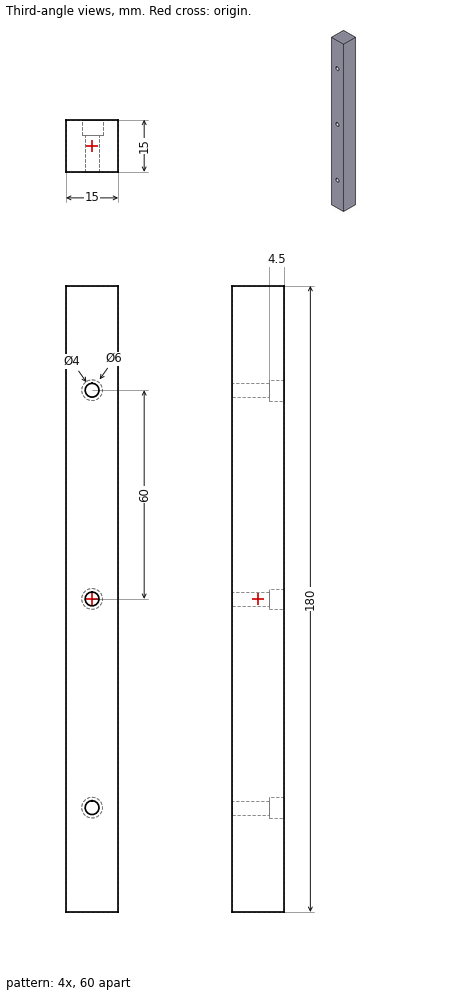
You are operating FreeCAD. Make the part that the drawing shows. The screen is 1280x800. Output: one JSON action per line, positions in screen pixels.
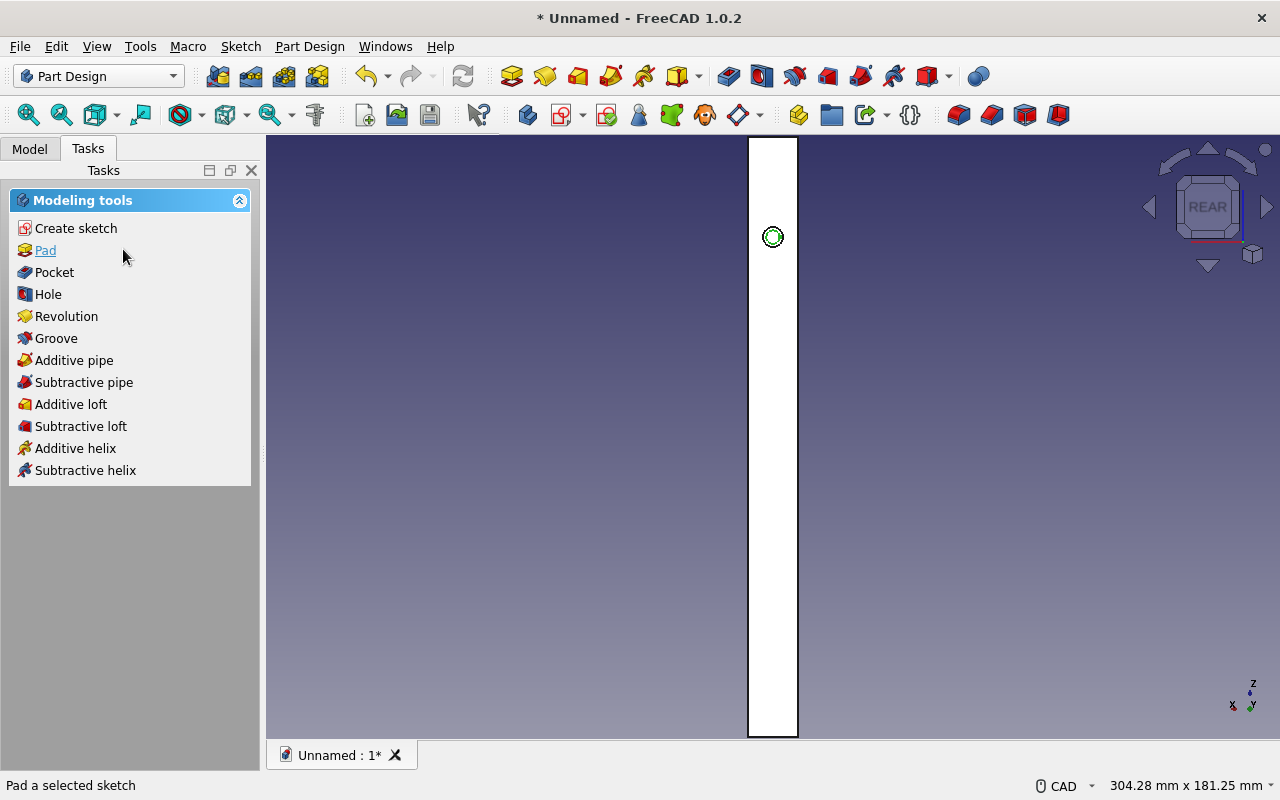
{"action": "left_click", "coordinate": [729, 76]}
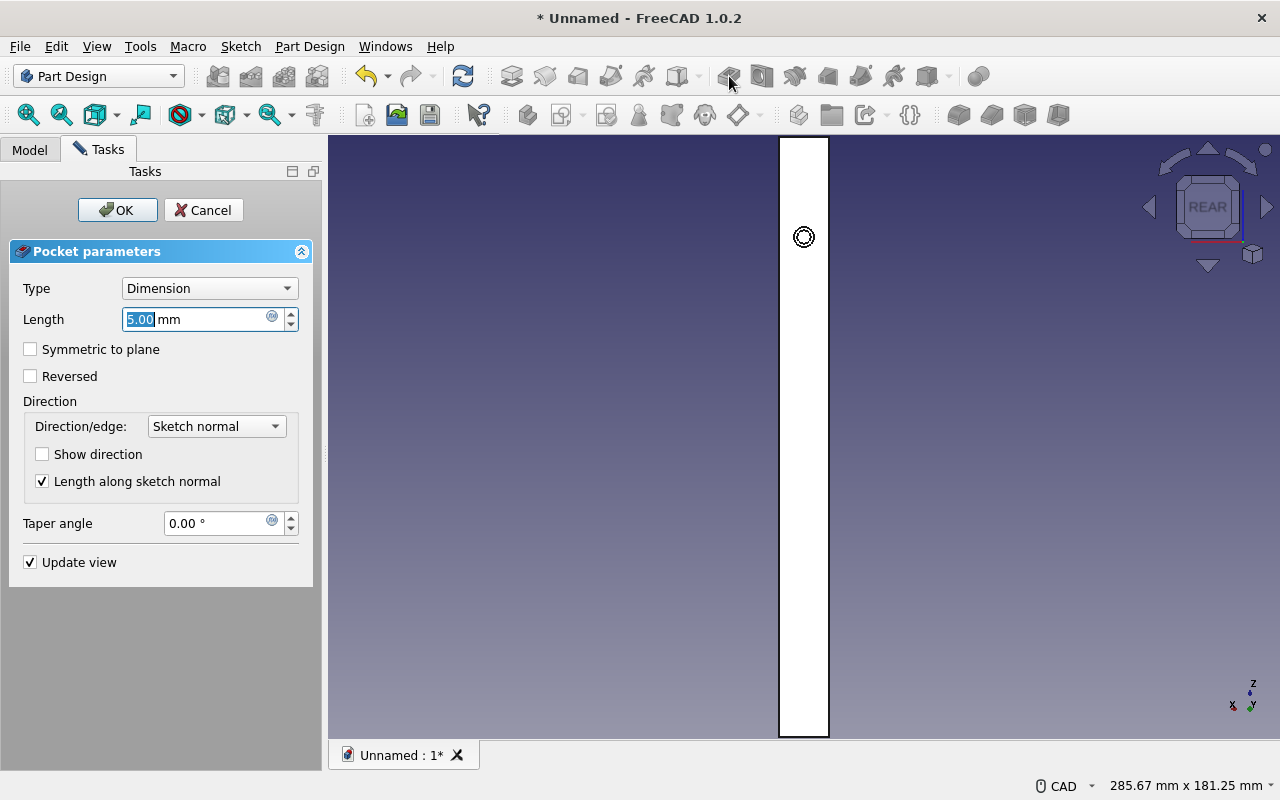
{"action": "left_click", "coordinate": [210, 288]}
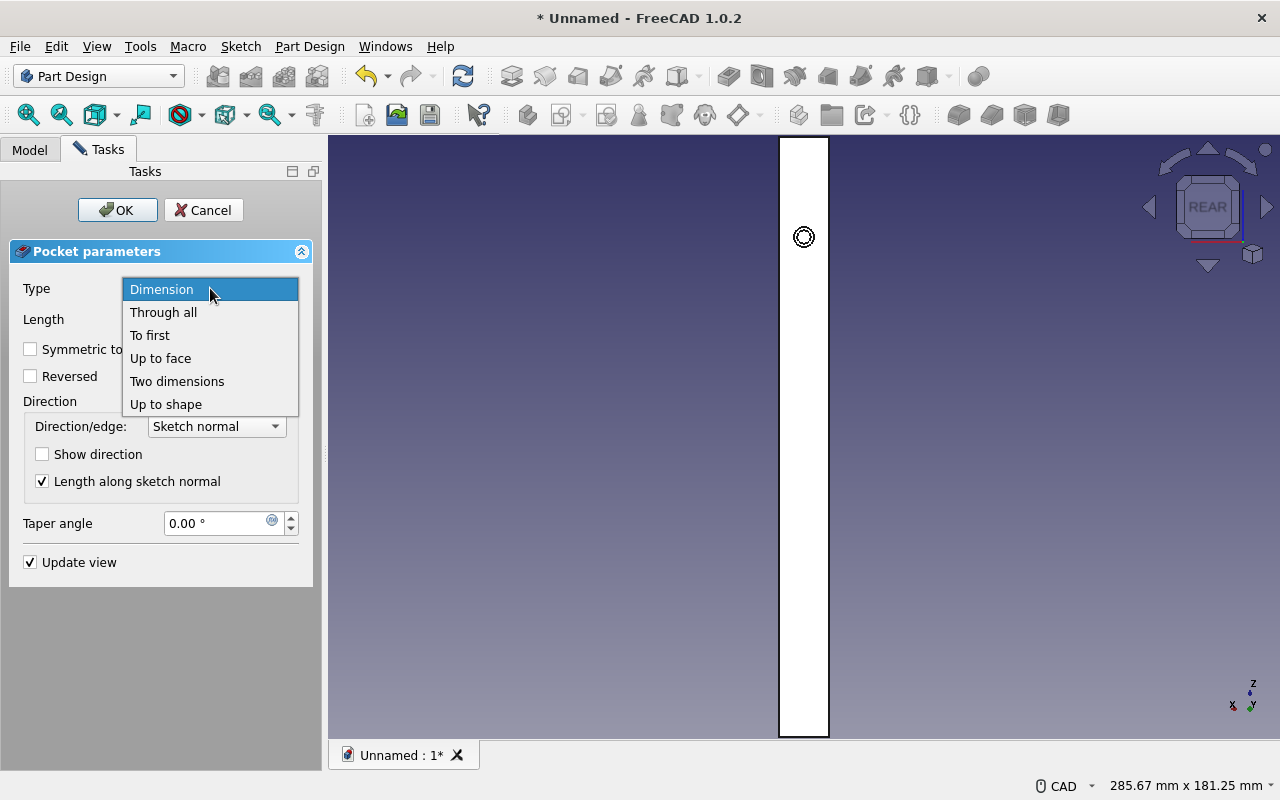
{"action": "left_click", "coordinate": [208, 312]}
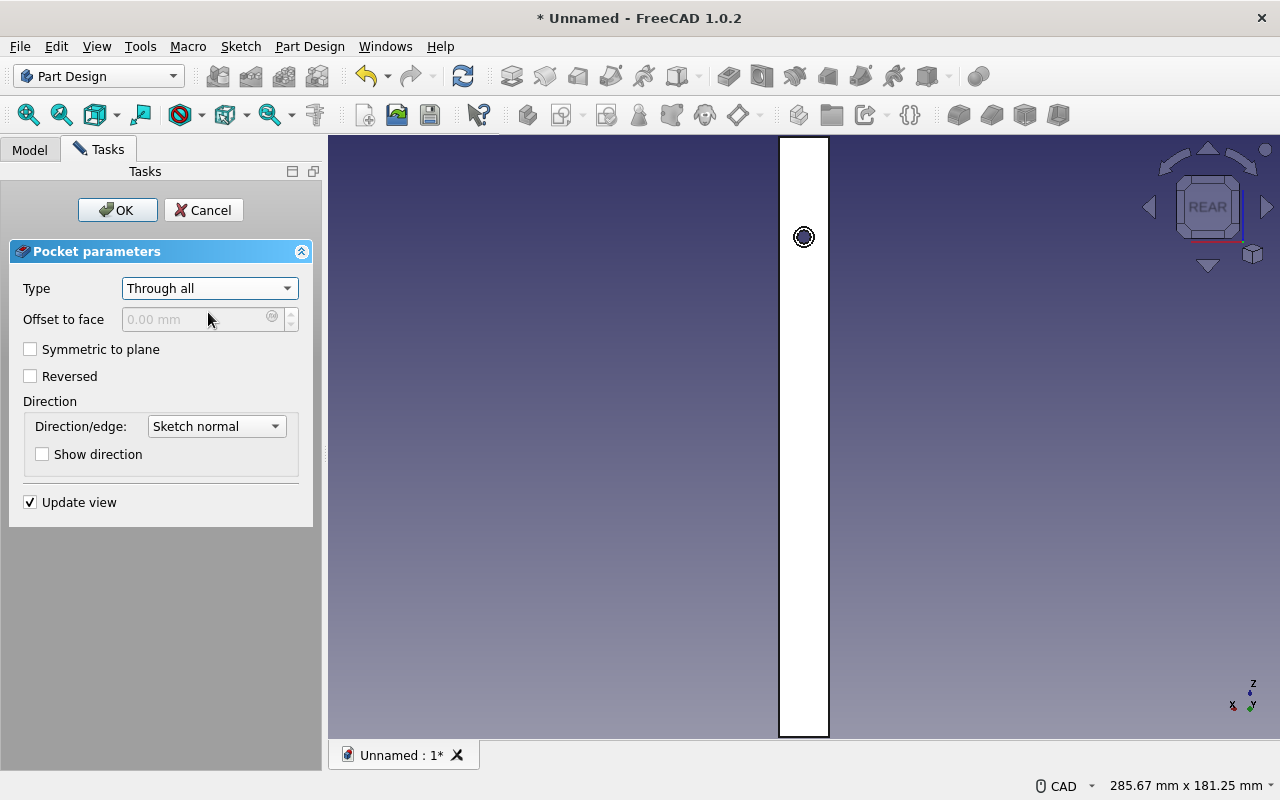
{"action": "left_click", "coordinate": [118, 210]}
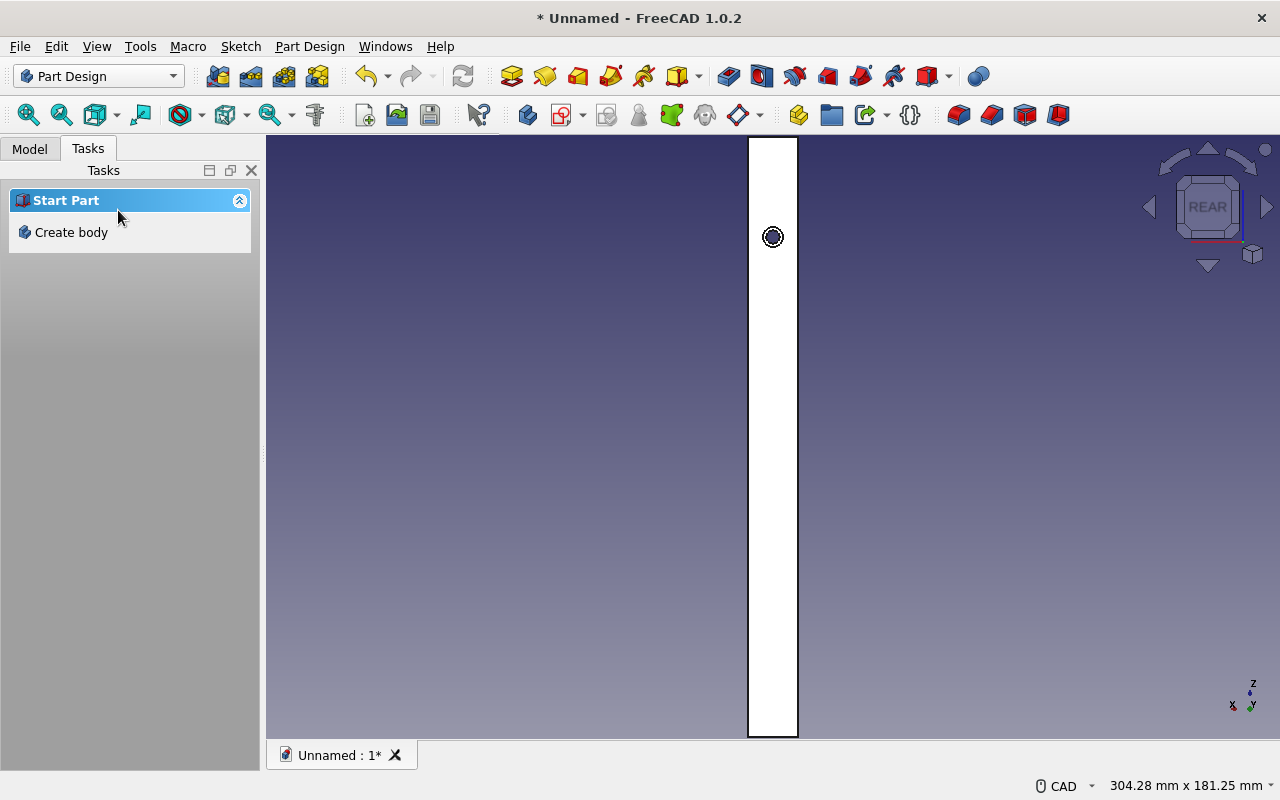
{"action": "left_click", "coordinate": [30, 148]}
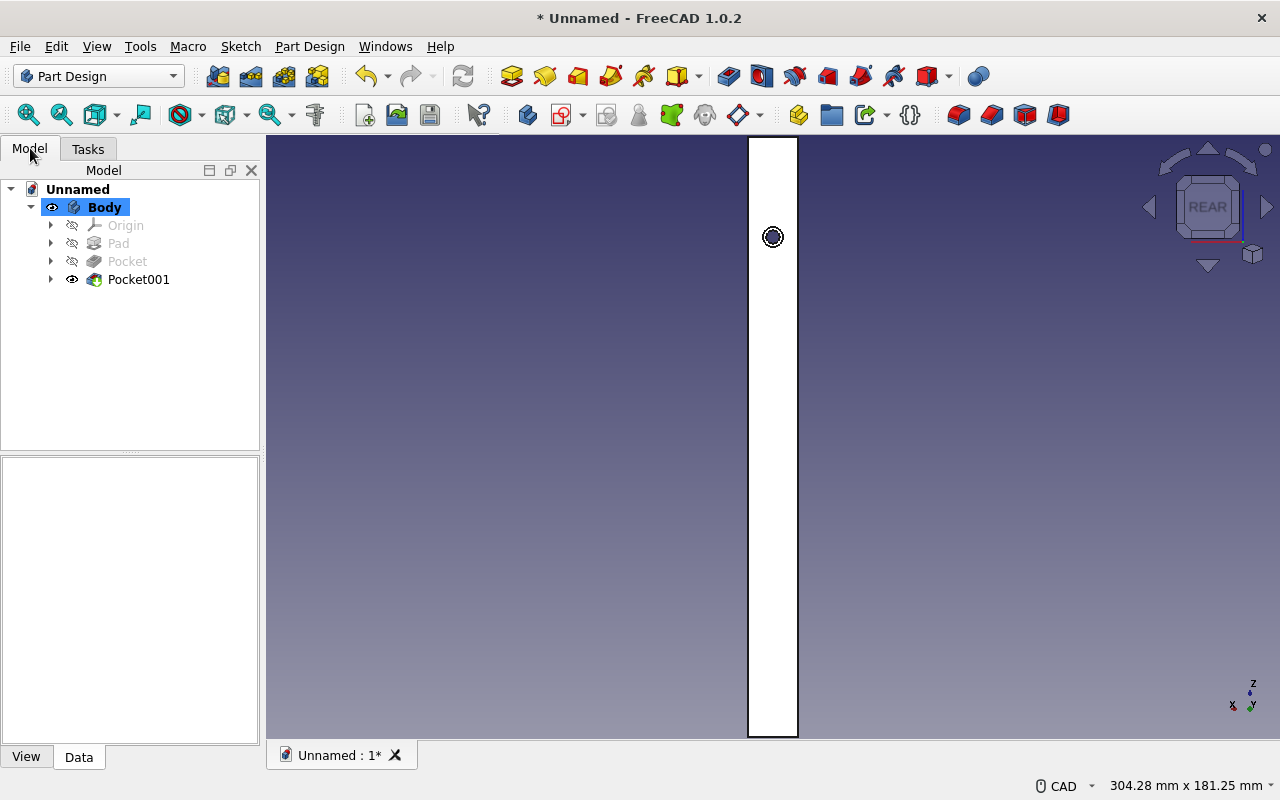
{"action": "left_click", "coordinate": [117, 261]}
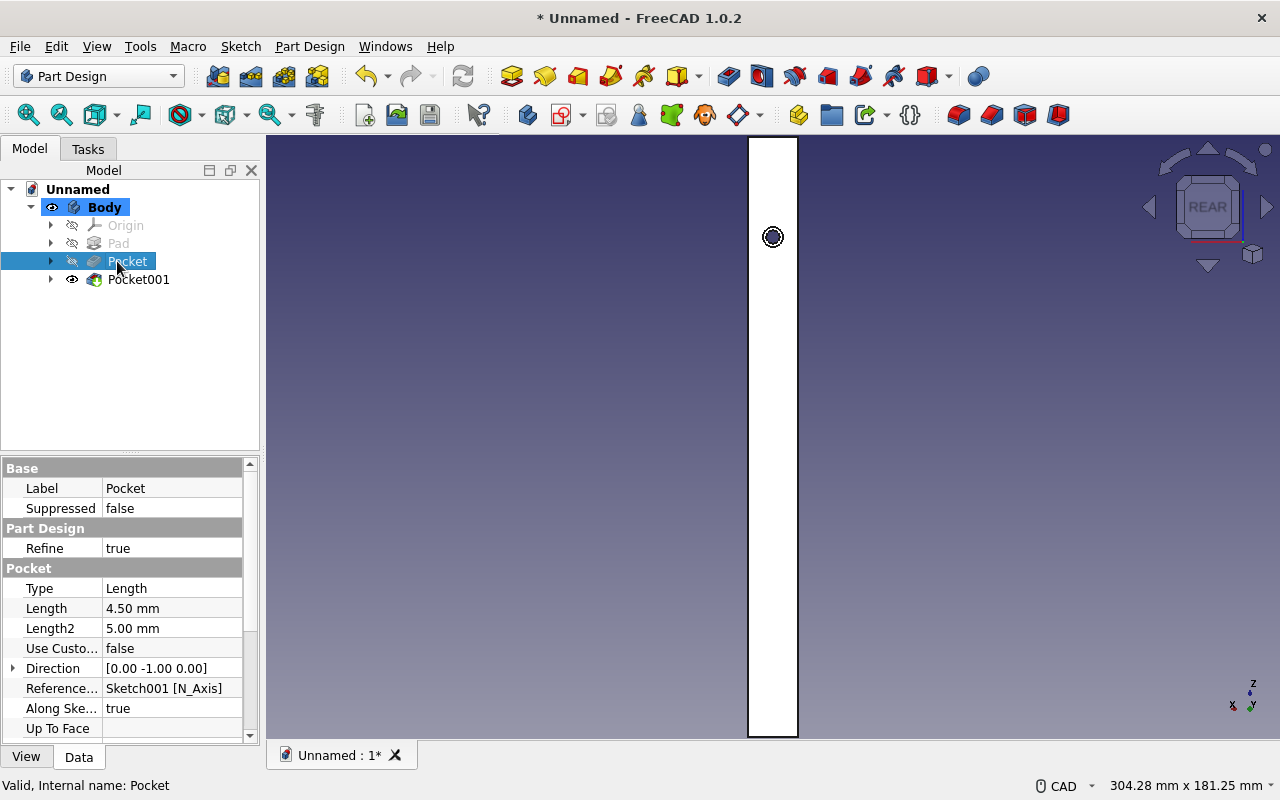
{"action": "left_click", "coordinate": [117, 279], "text": "ctrl"}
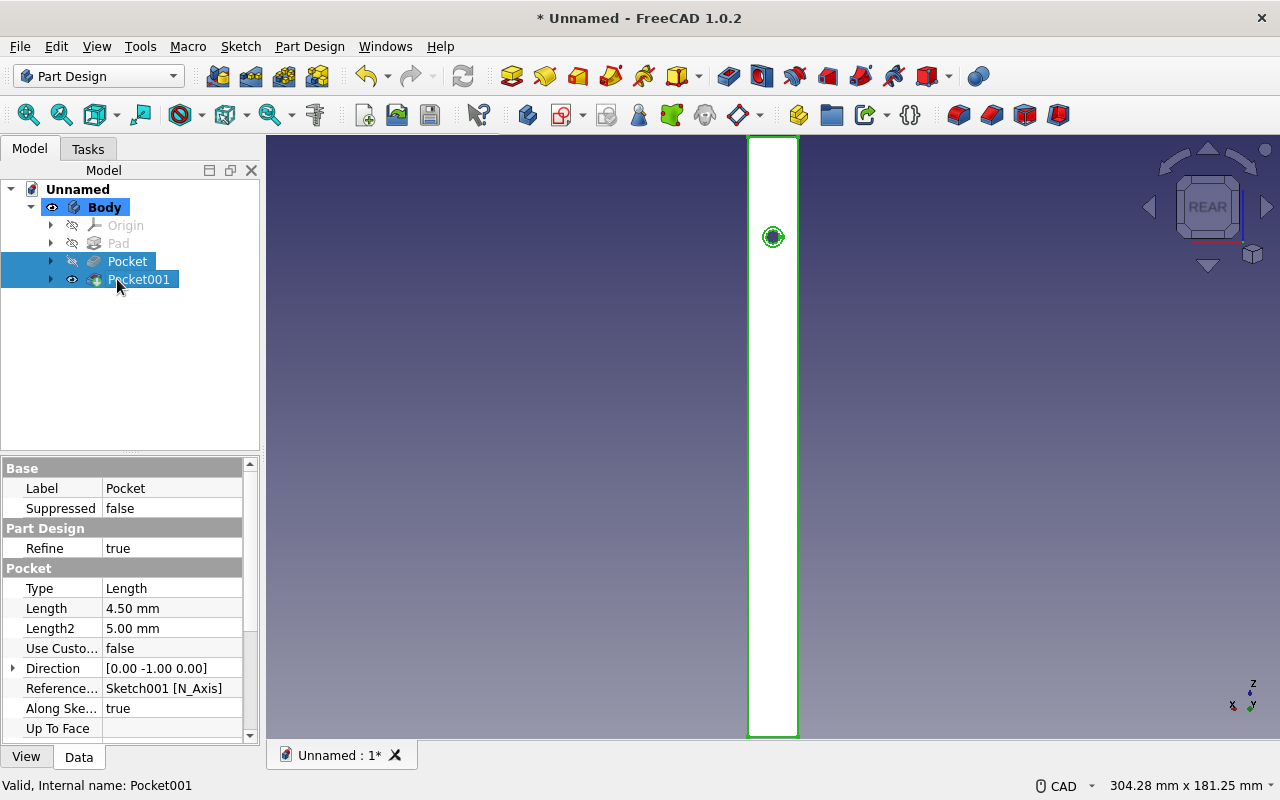
{"action": "left_click", "coordinate": [251, 76]}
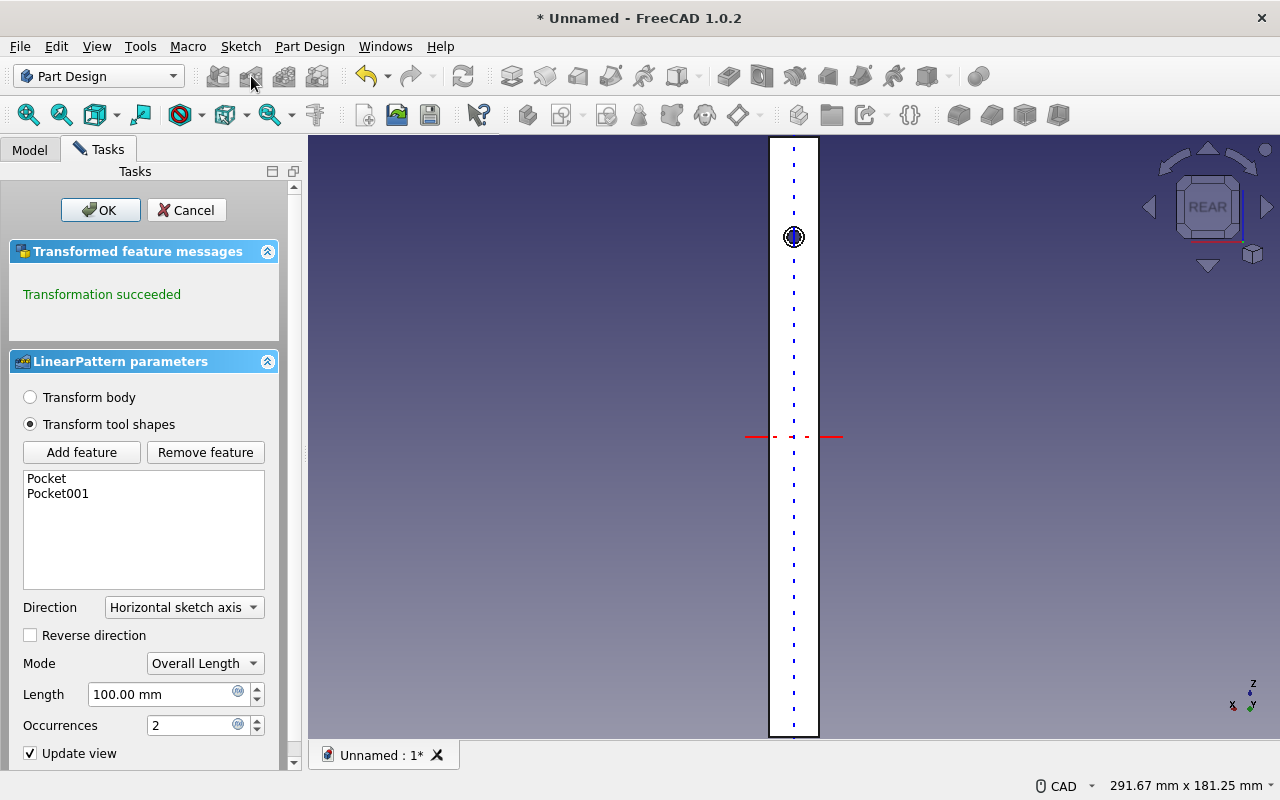
{"action": "left_click", "coordinate": [185, 608]}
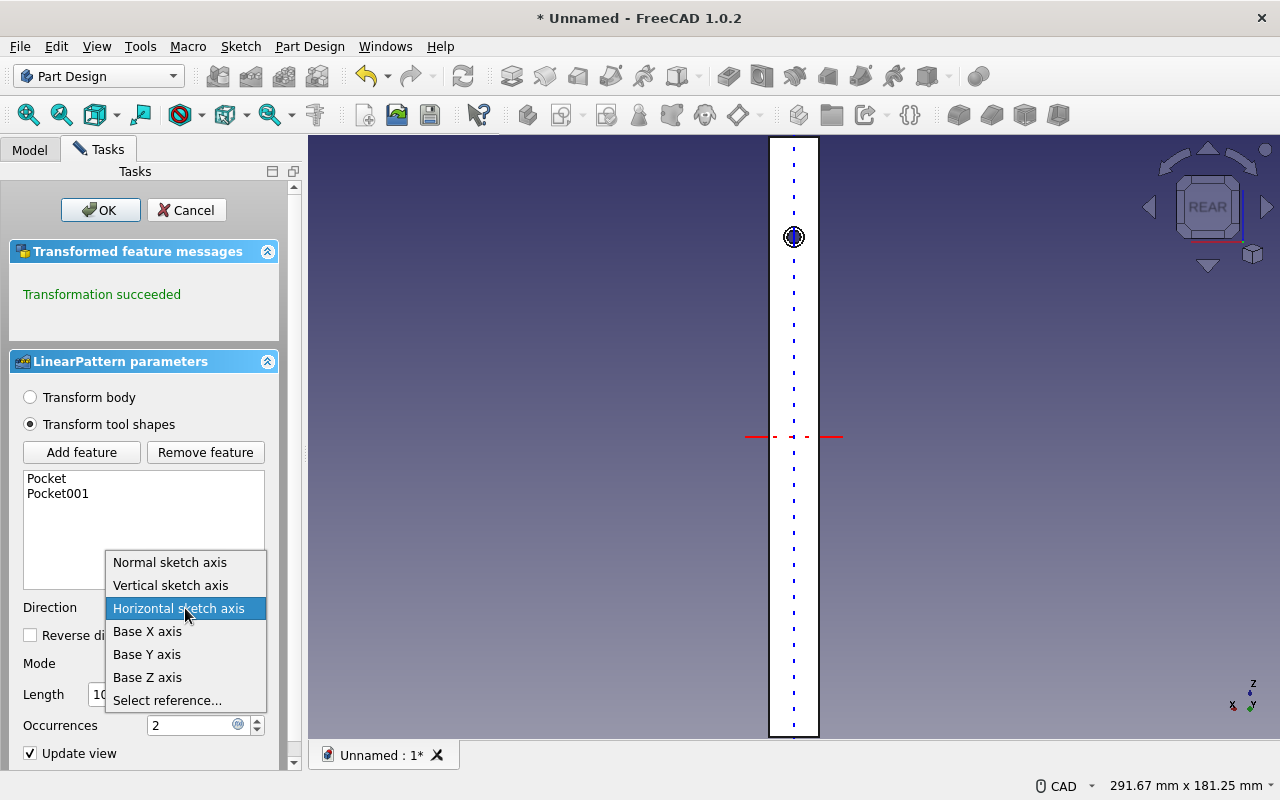
{"action": "left_click", "coordinate": [184, 678]}